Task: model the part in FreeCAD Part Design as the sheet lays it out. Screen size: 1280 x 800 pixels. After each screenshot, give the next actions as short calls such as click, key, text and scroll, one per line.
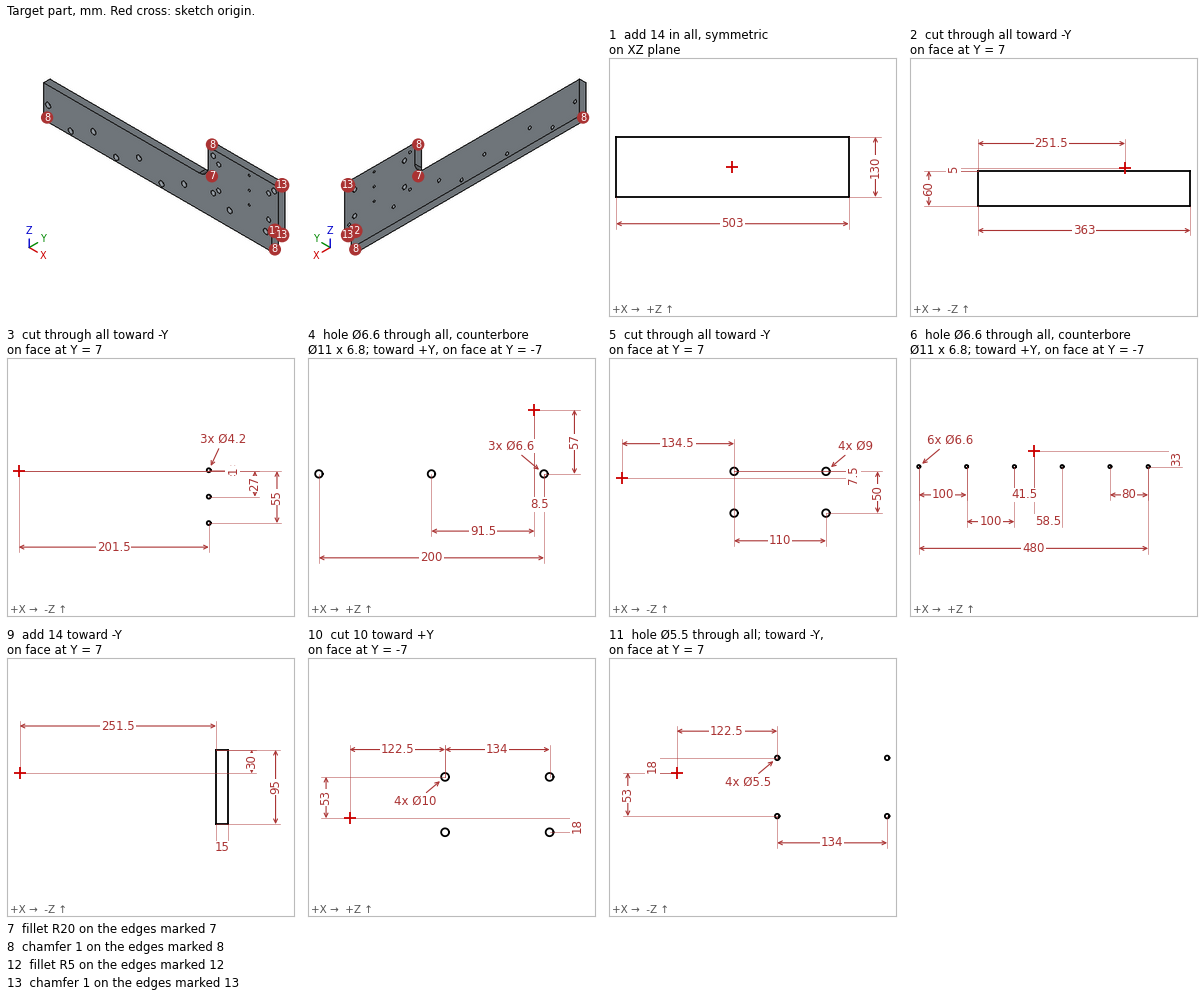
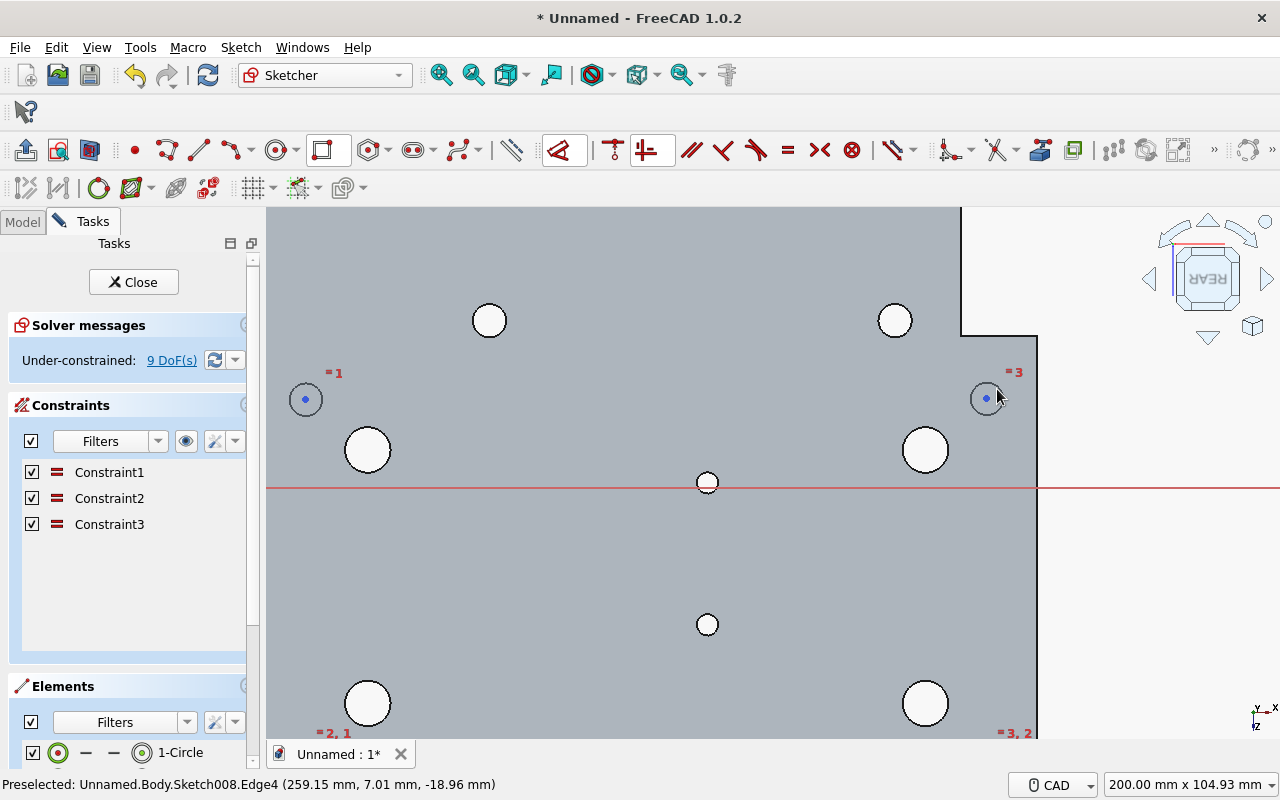
click(306, 400)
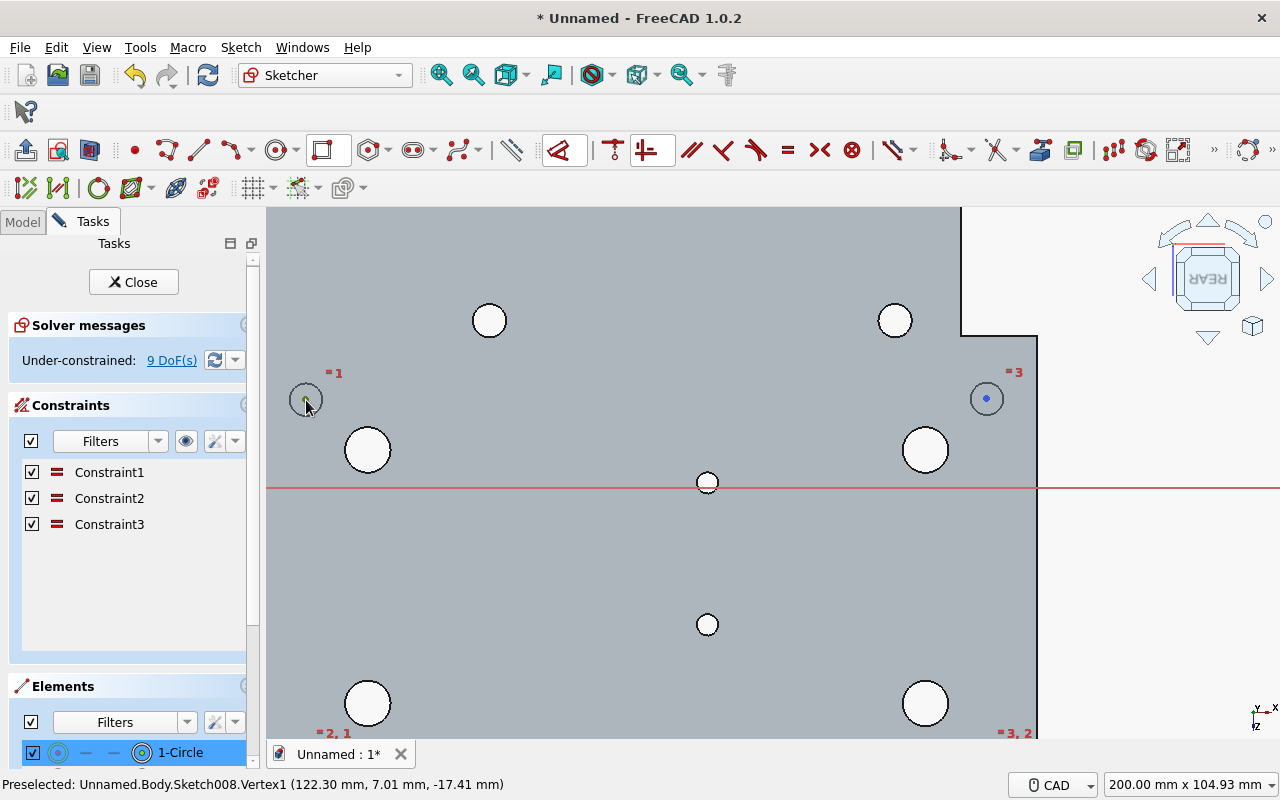
scroll(999, 388, down, 4)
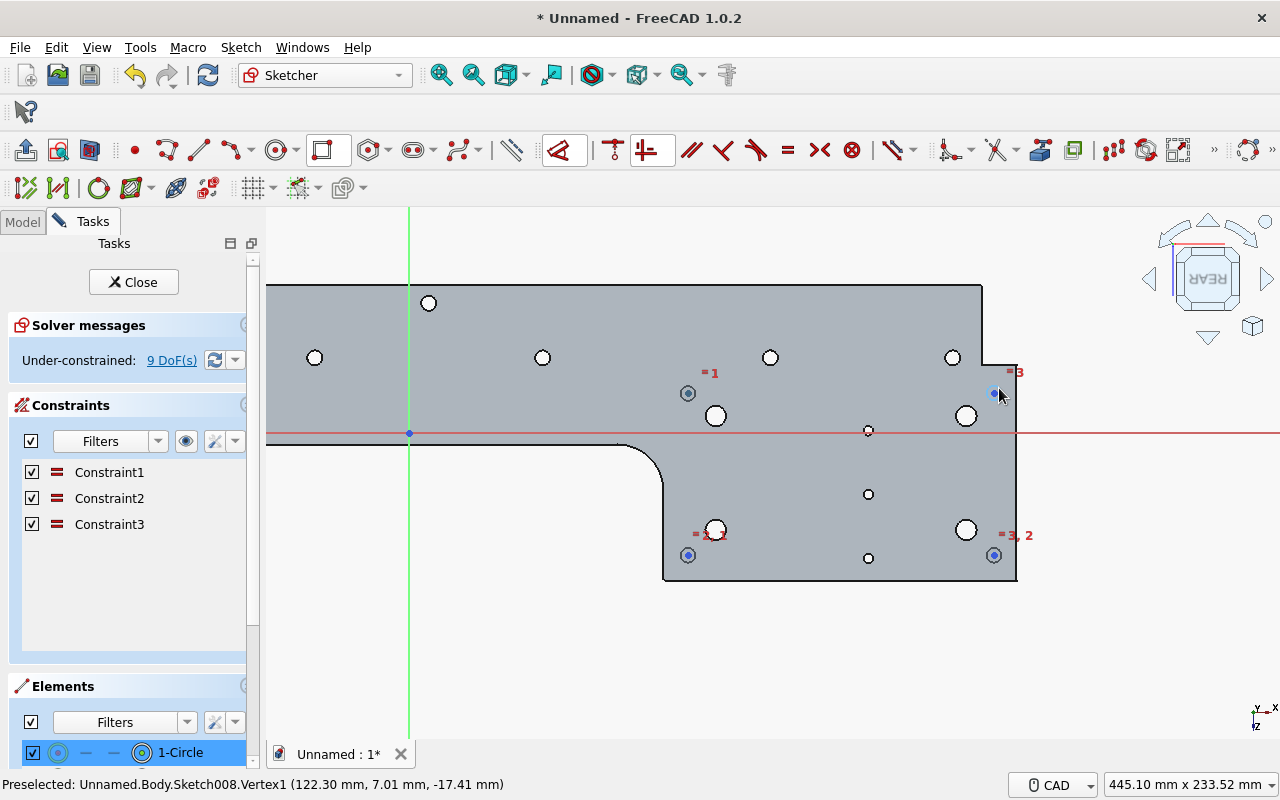
click(688, 555)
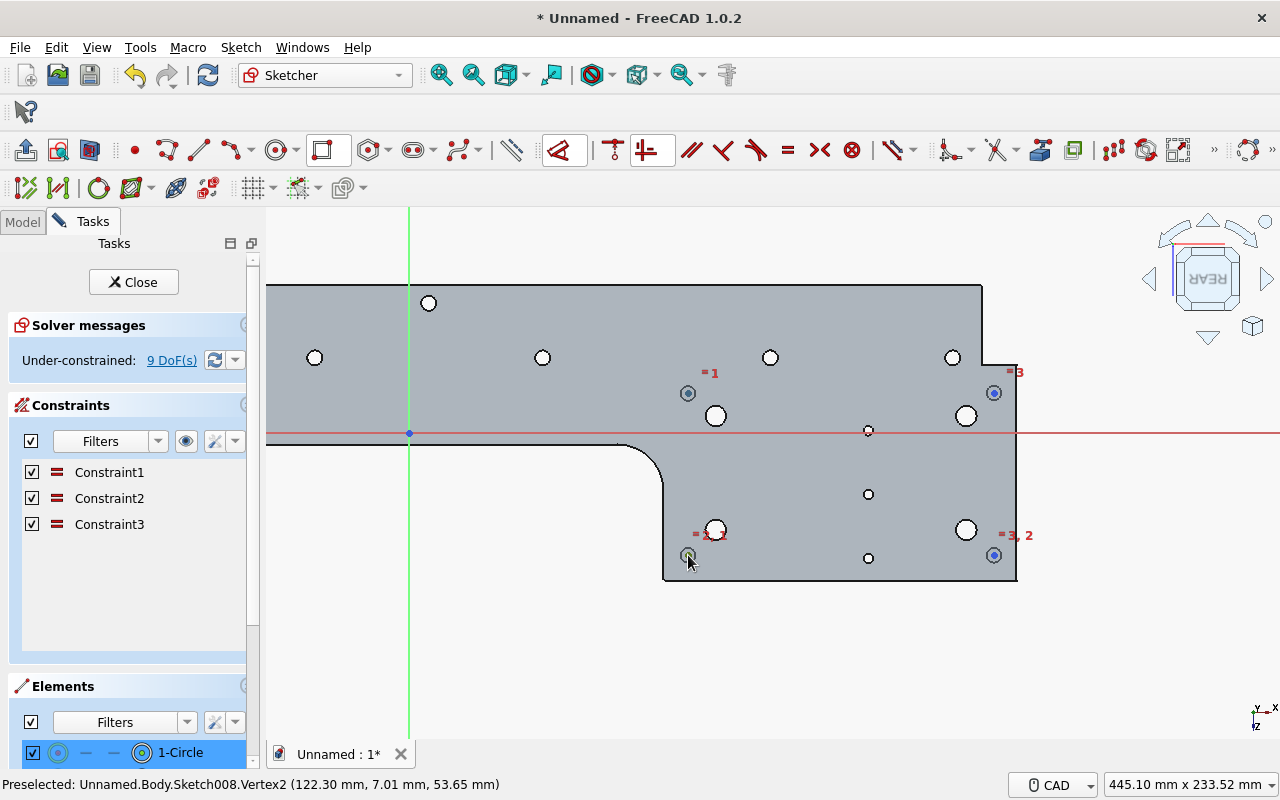
key(v)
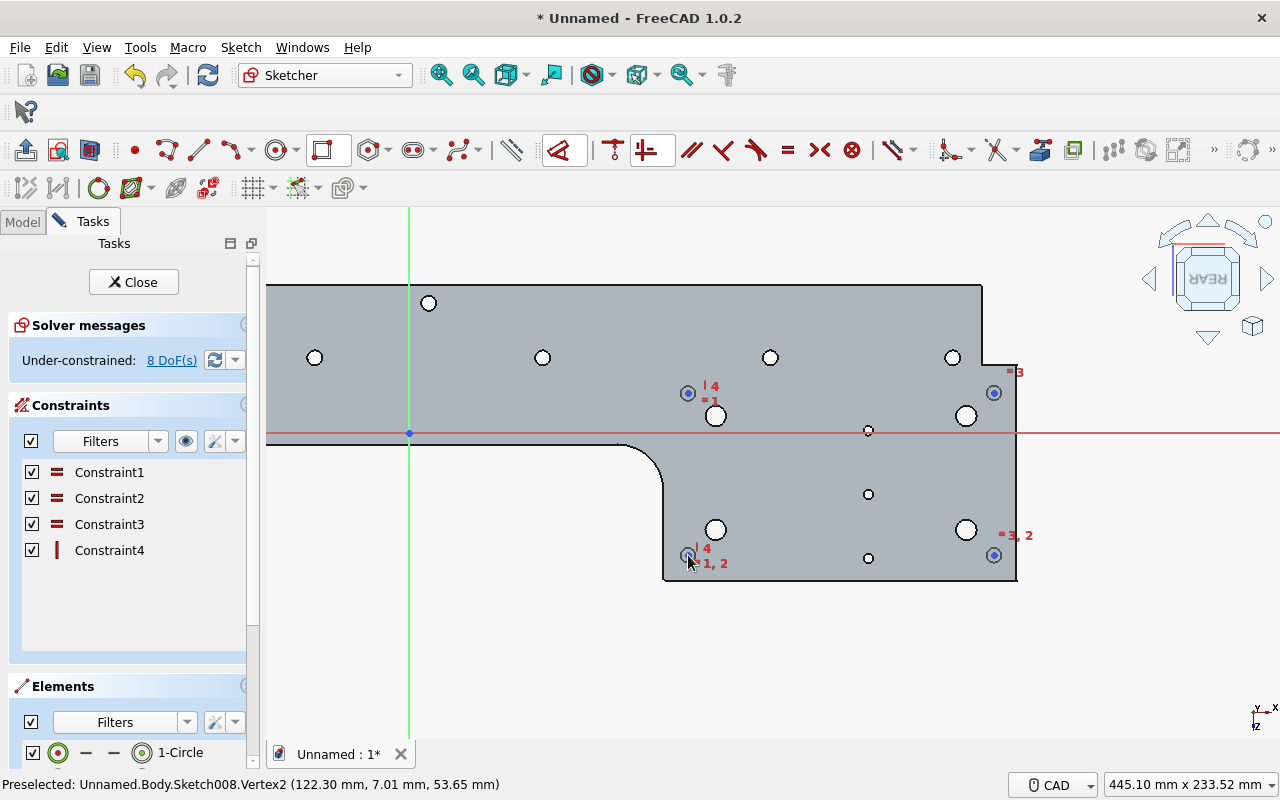
click(688, 555)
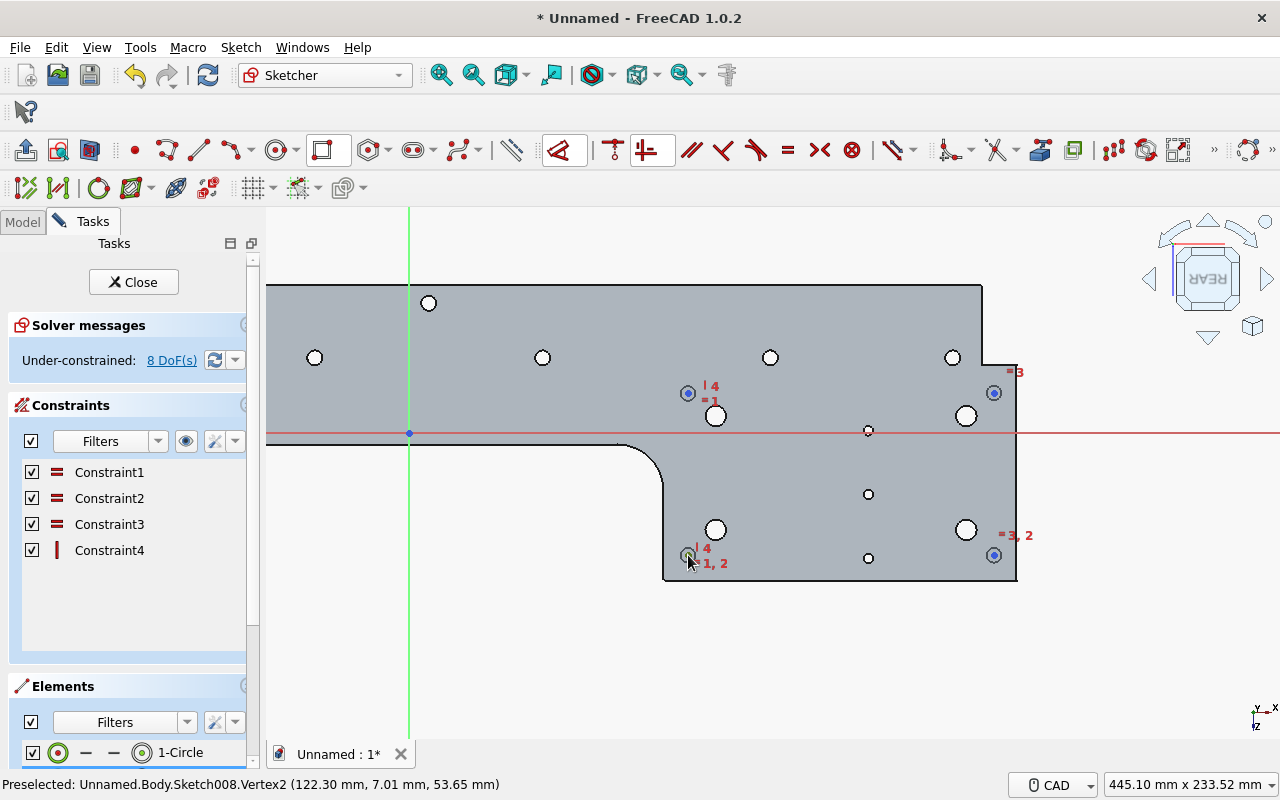
click(994, 555)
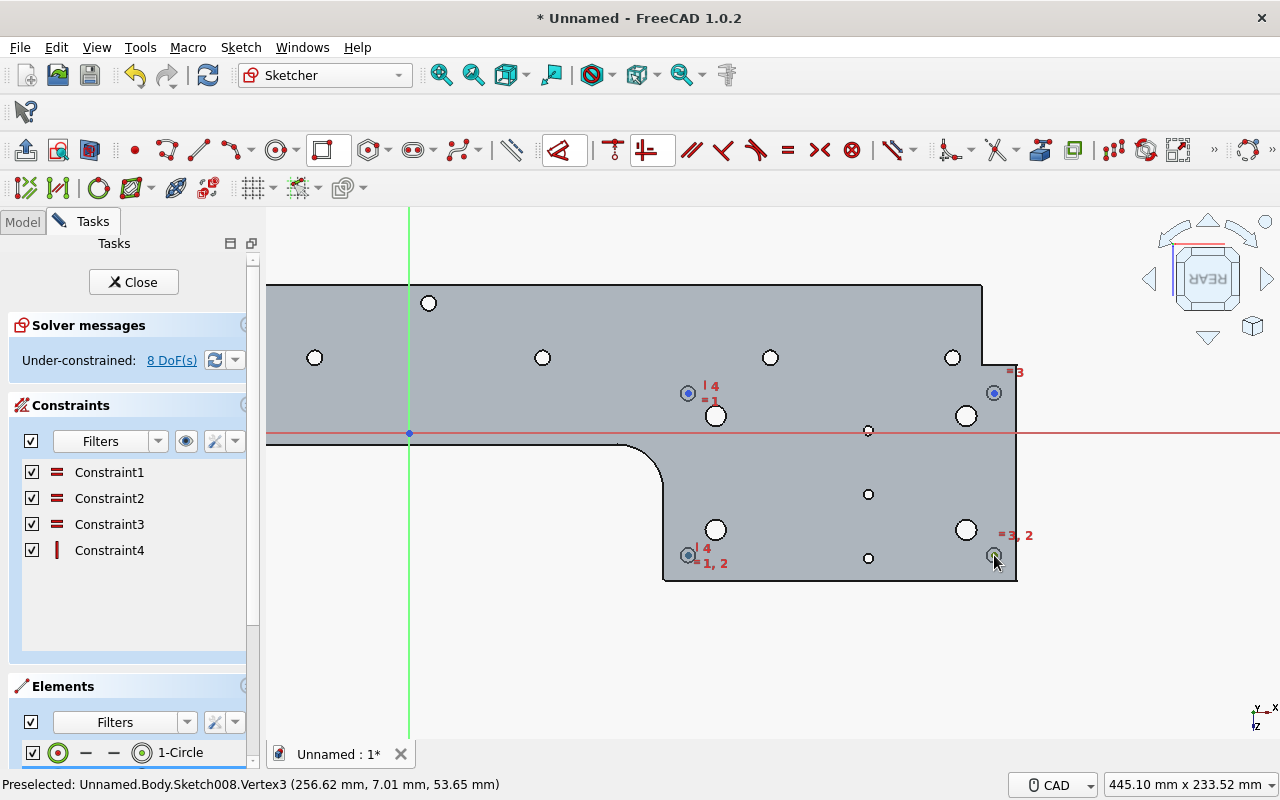
click(670, 150)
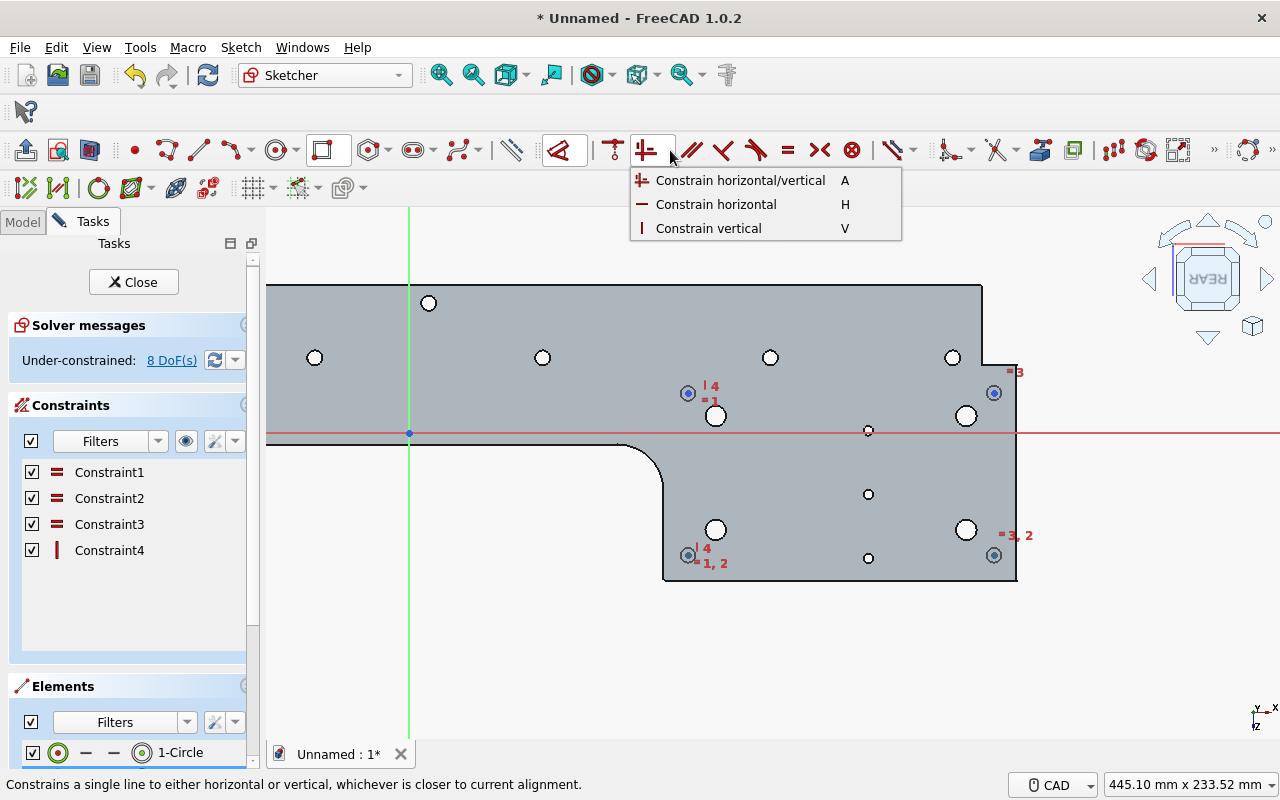
click(766, 204)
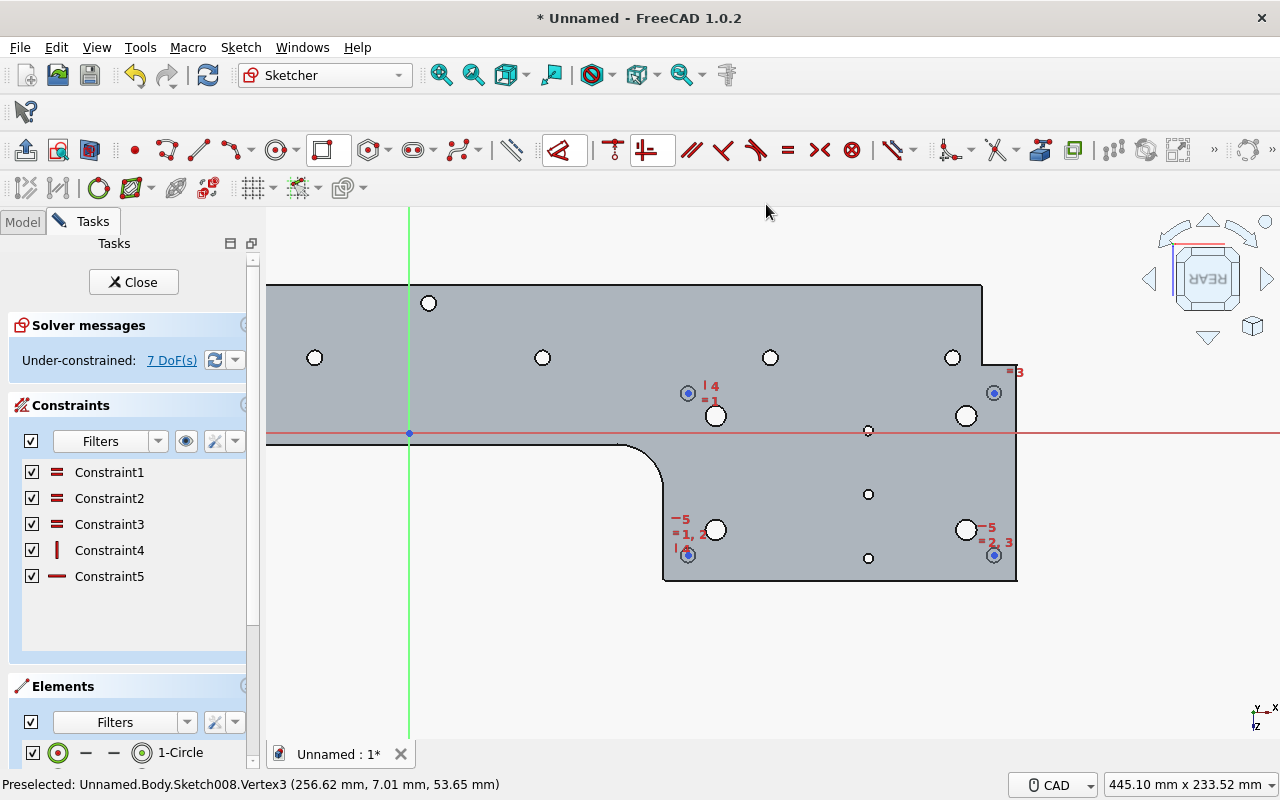
click(994, 555)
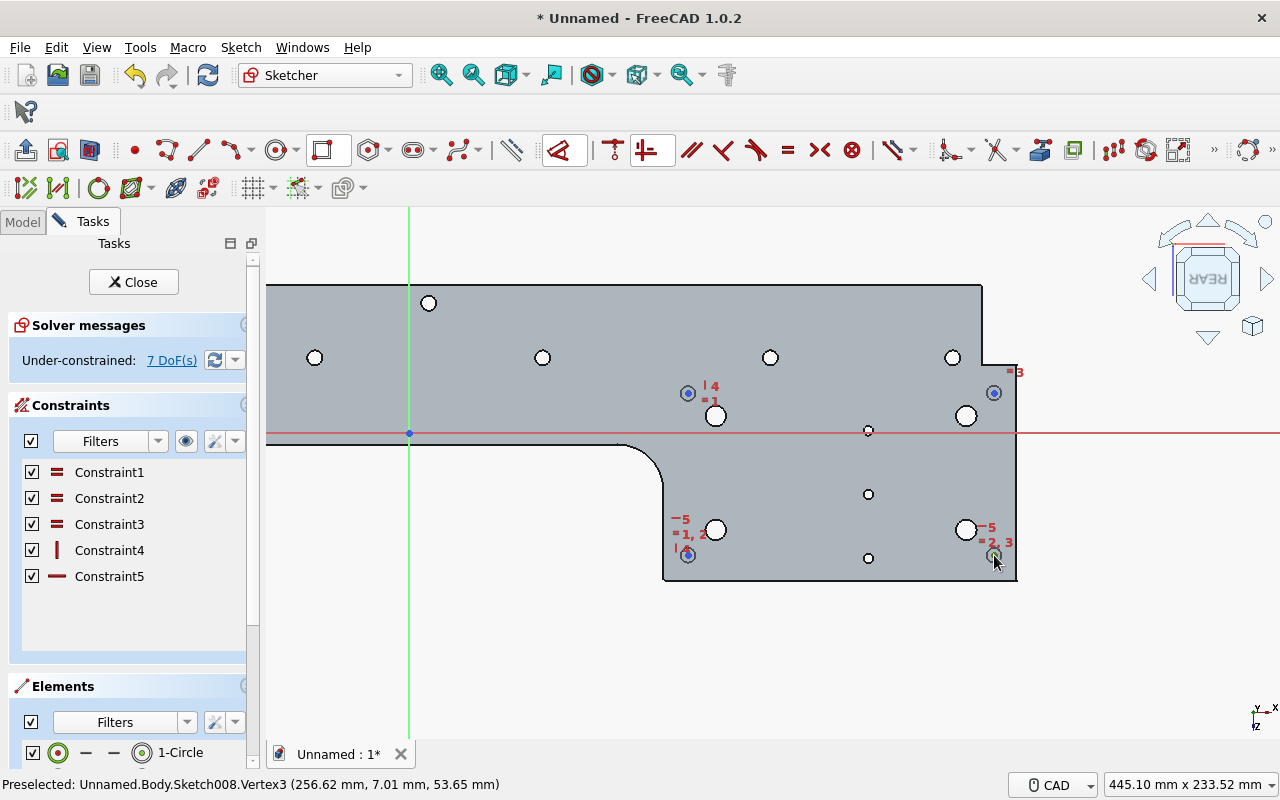
click(994, 393)